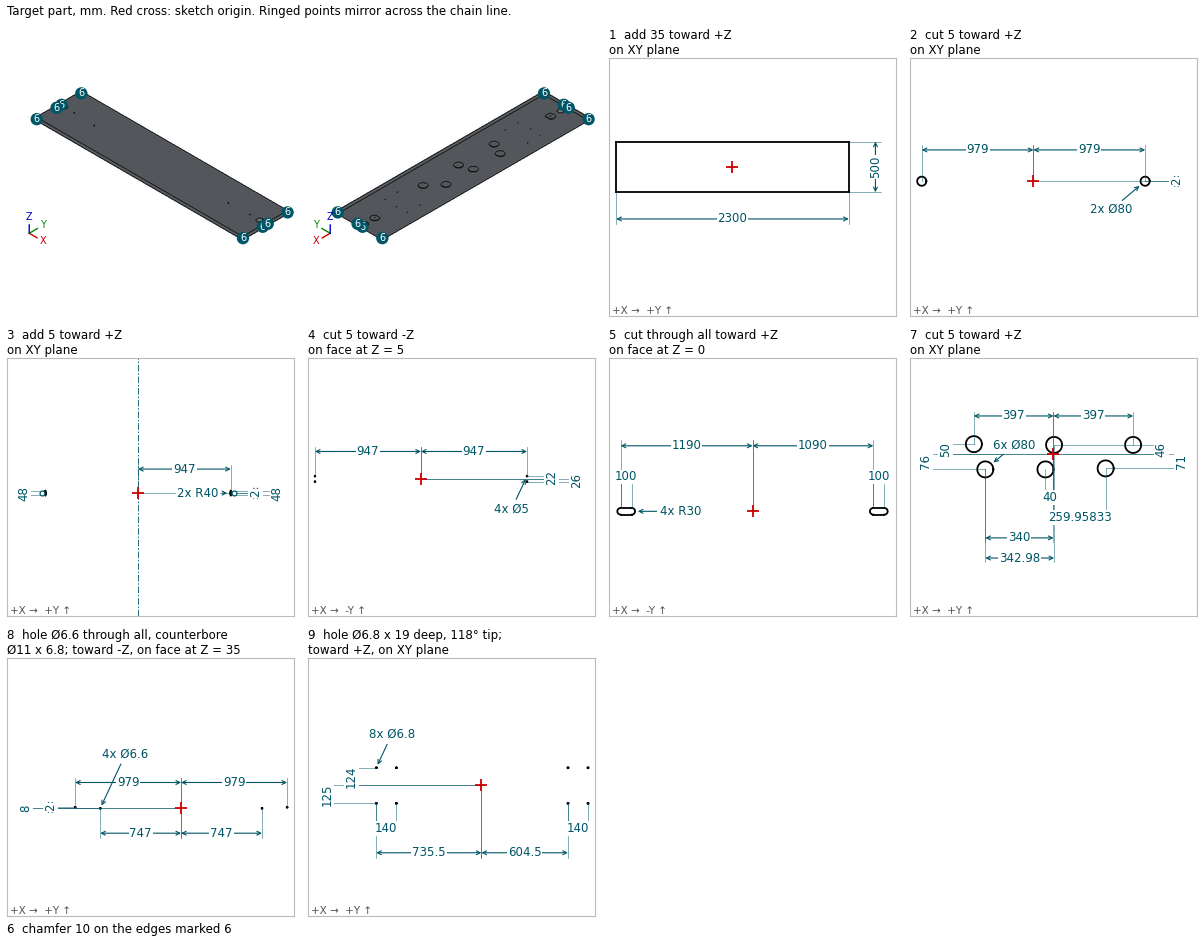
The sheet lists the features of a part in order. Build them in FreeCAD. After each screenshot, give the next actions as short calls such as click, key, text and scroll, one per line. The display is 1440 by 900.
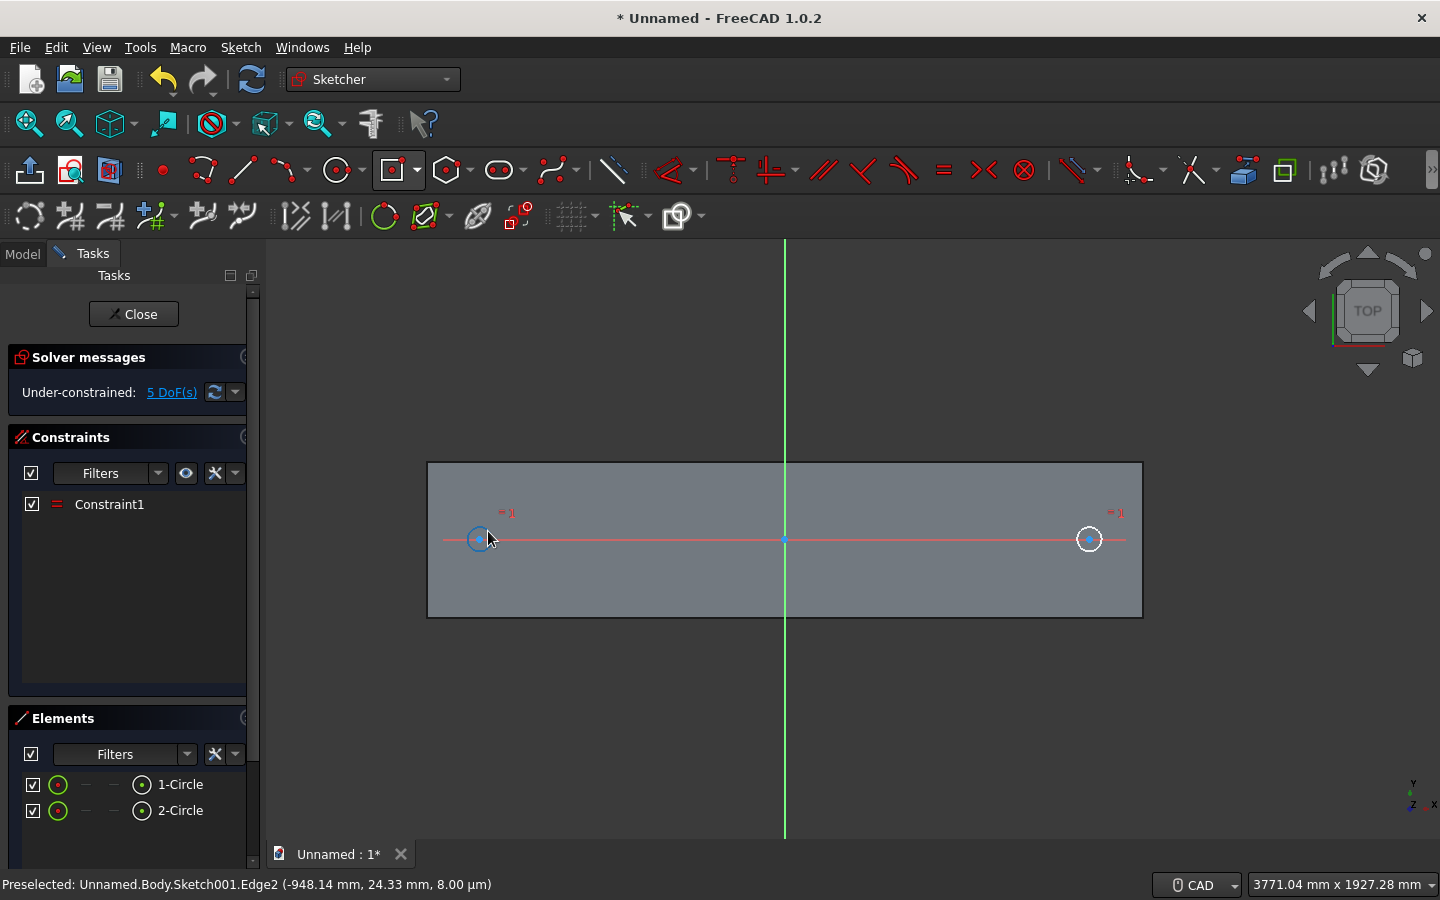
click(1089, 539)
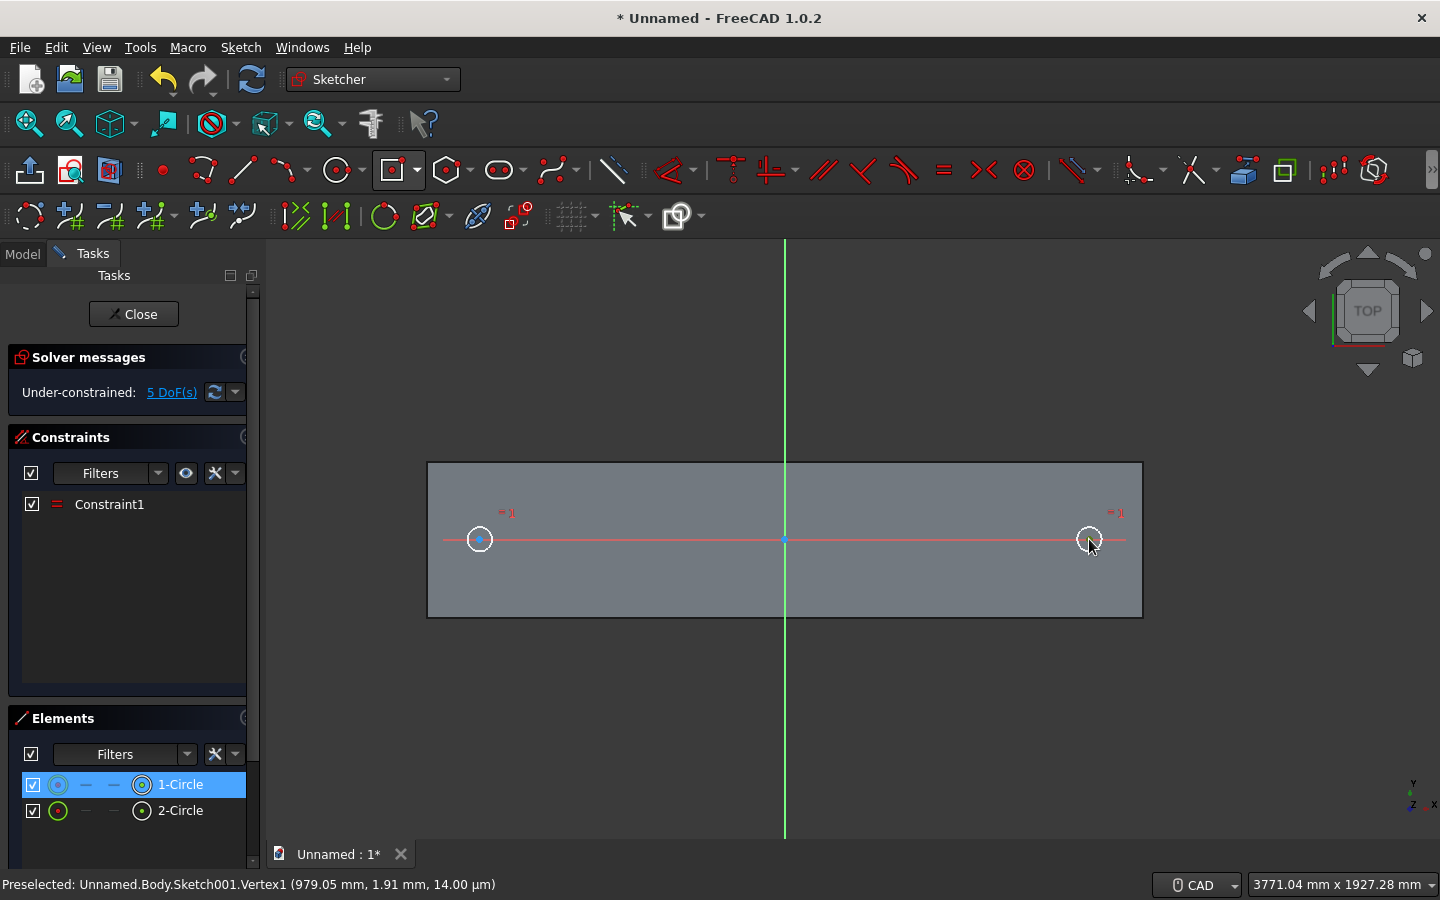
click(480, 539)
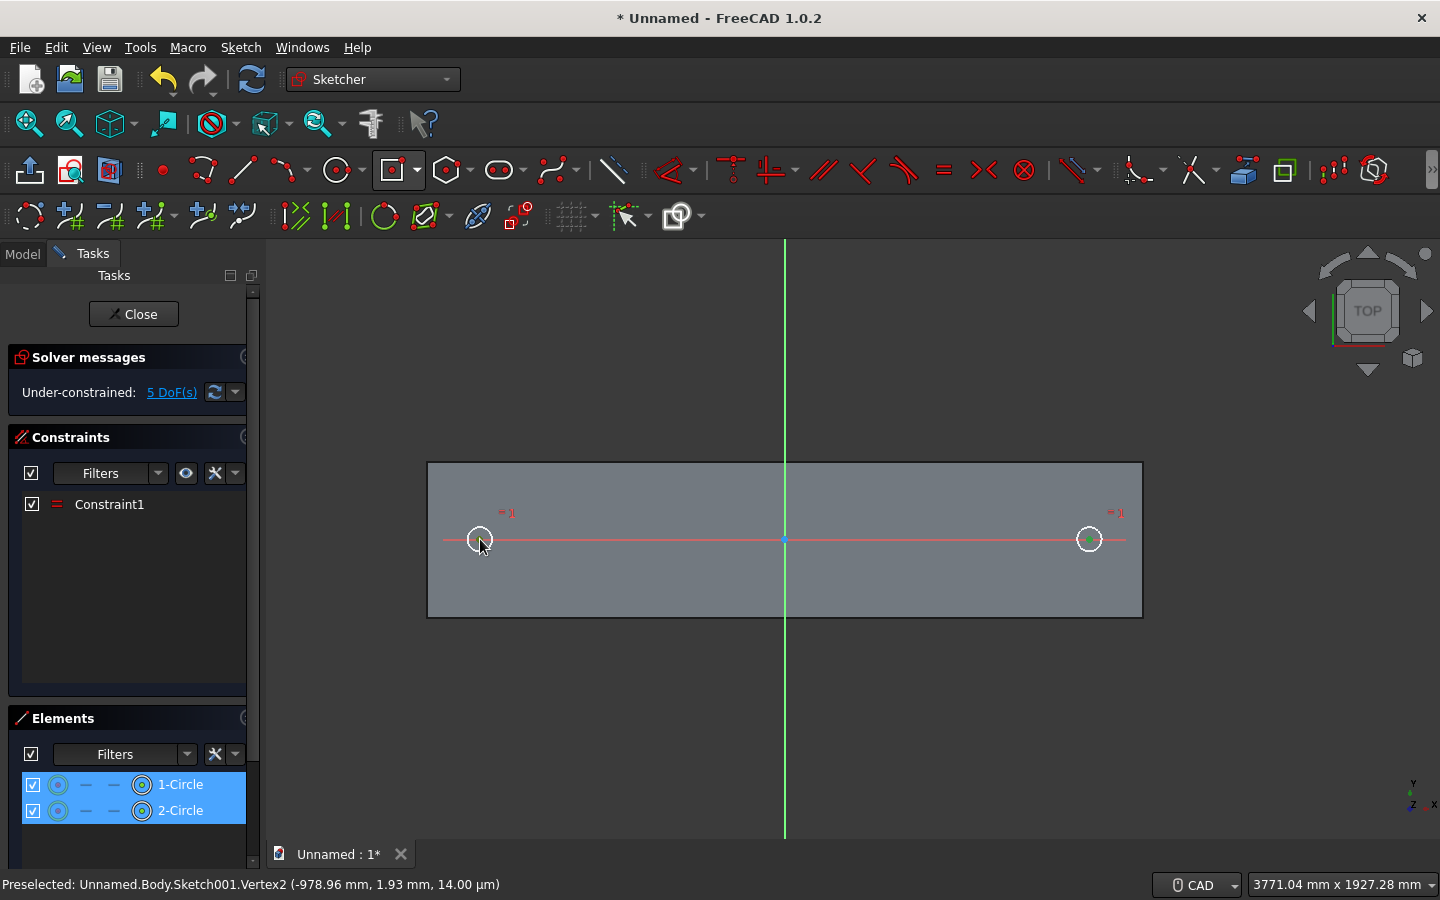
key(h)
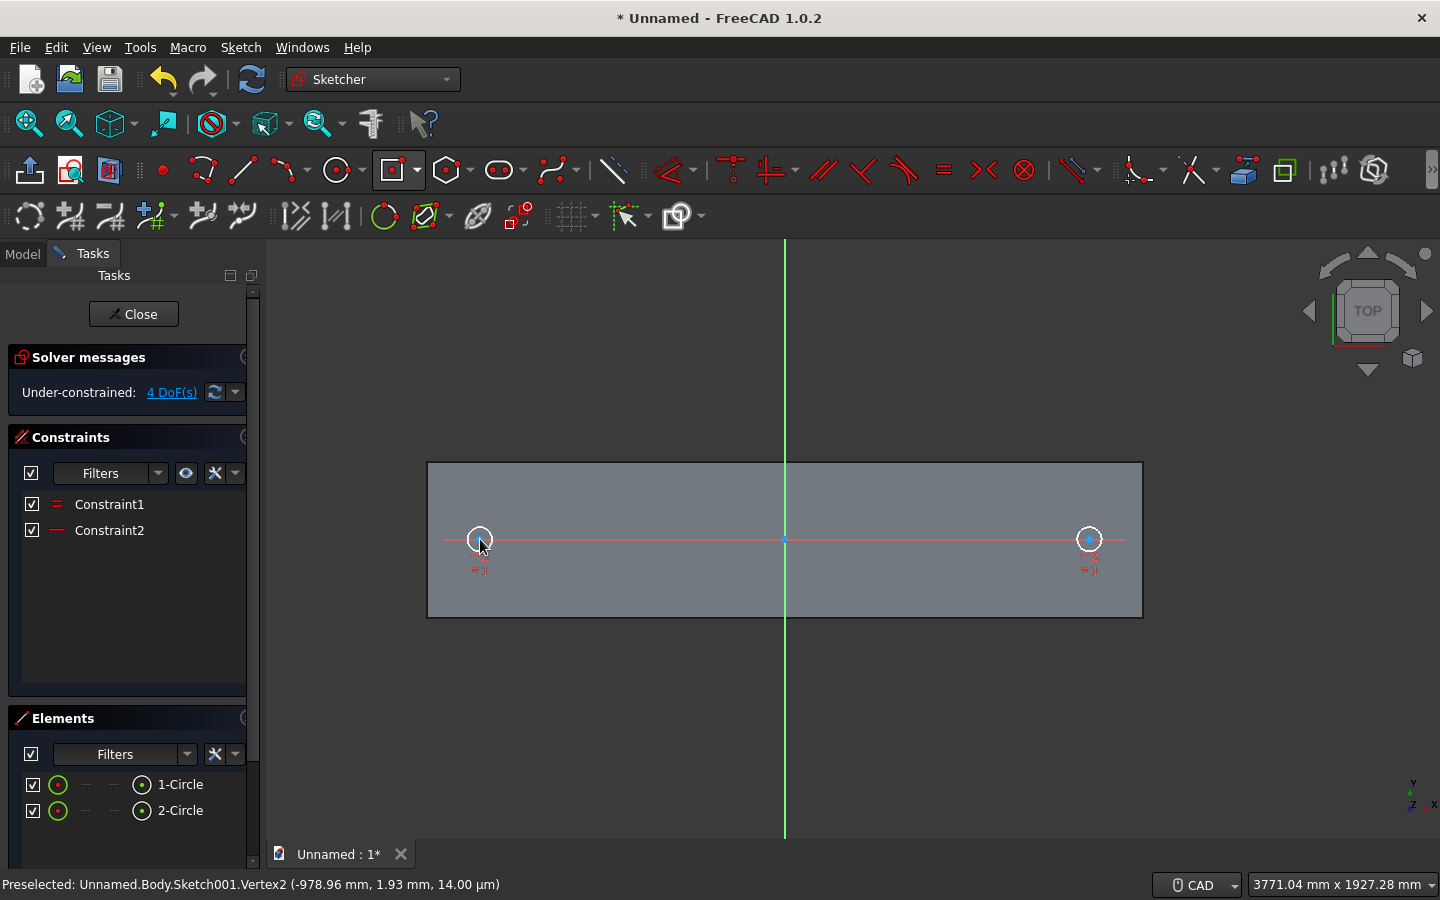
click(668, 170)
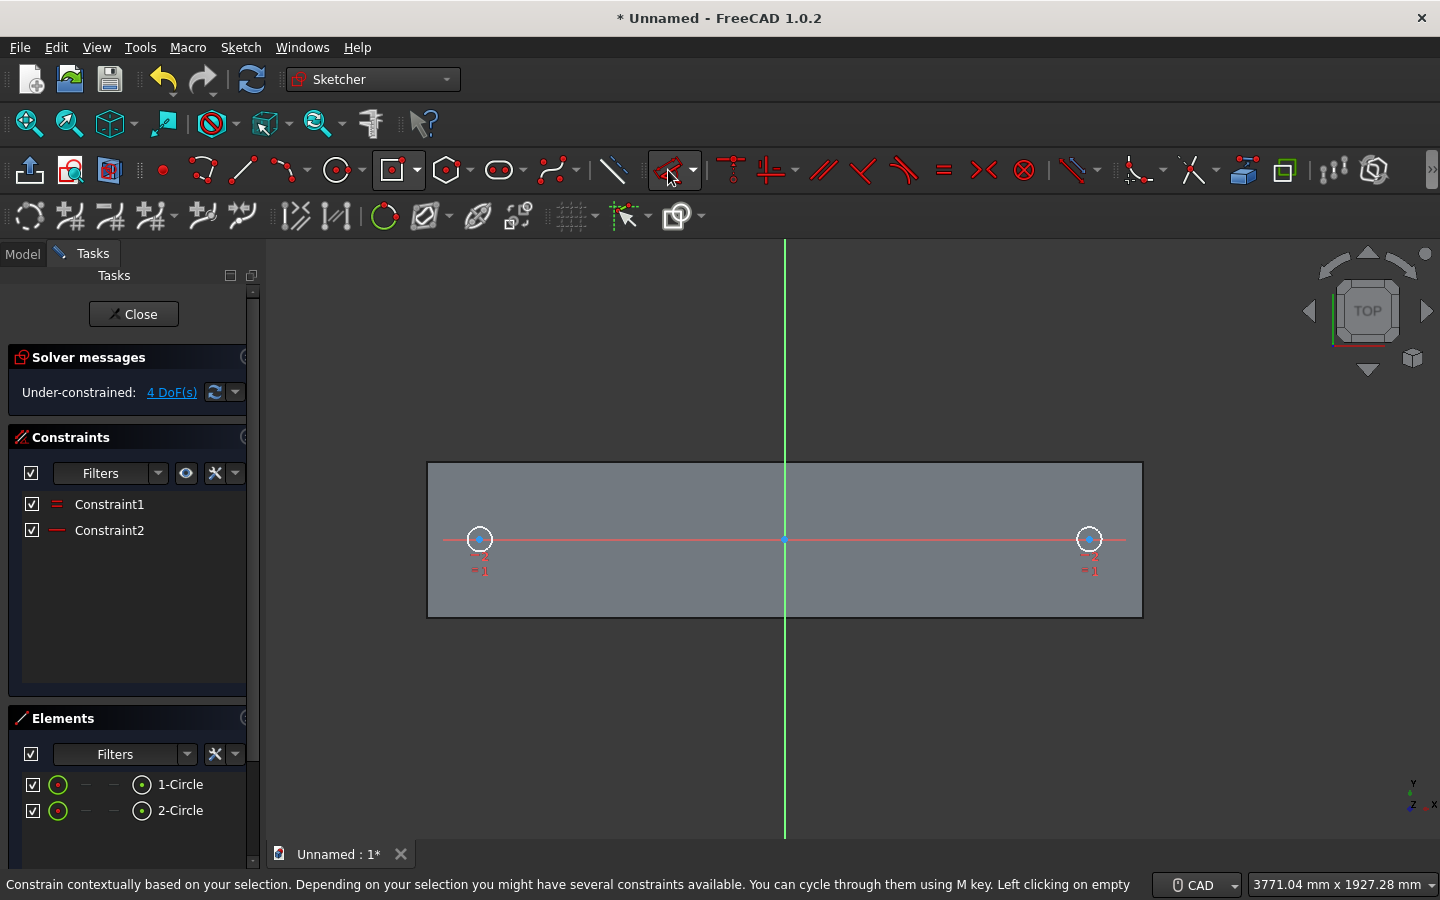
scroll(1098, 531, up, 3)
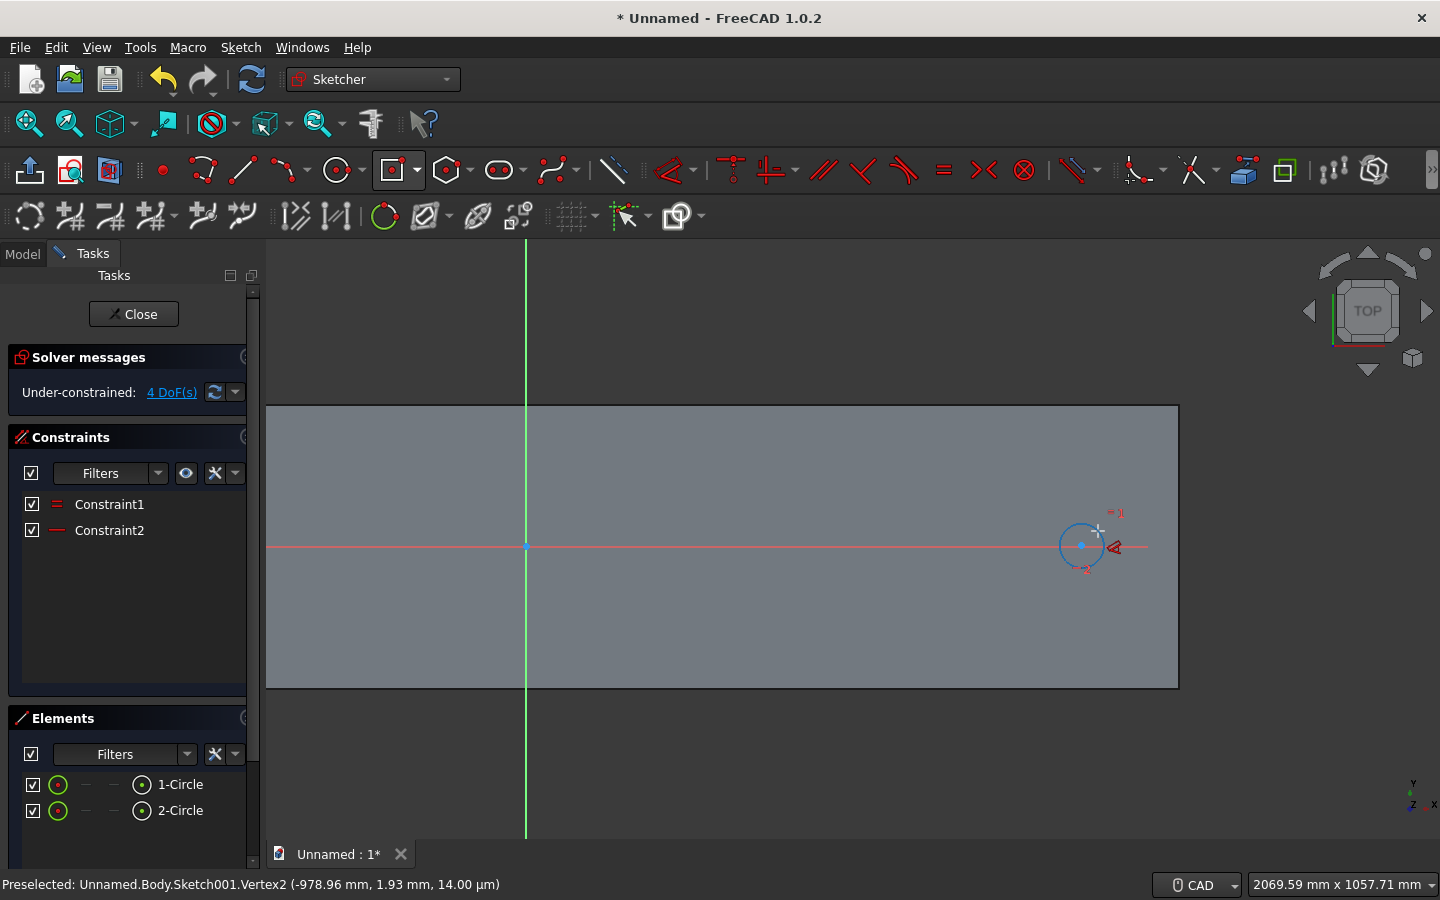
click(1097, 530)
click(1119, 507)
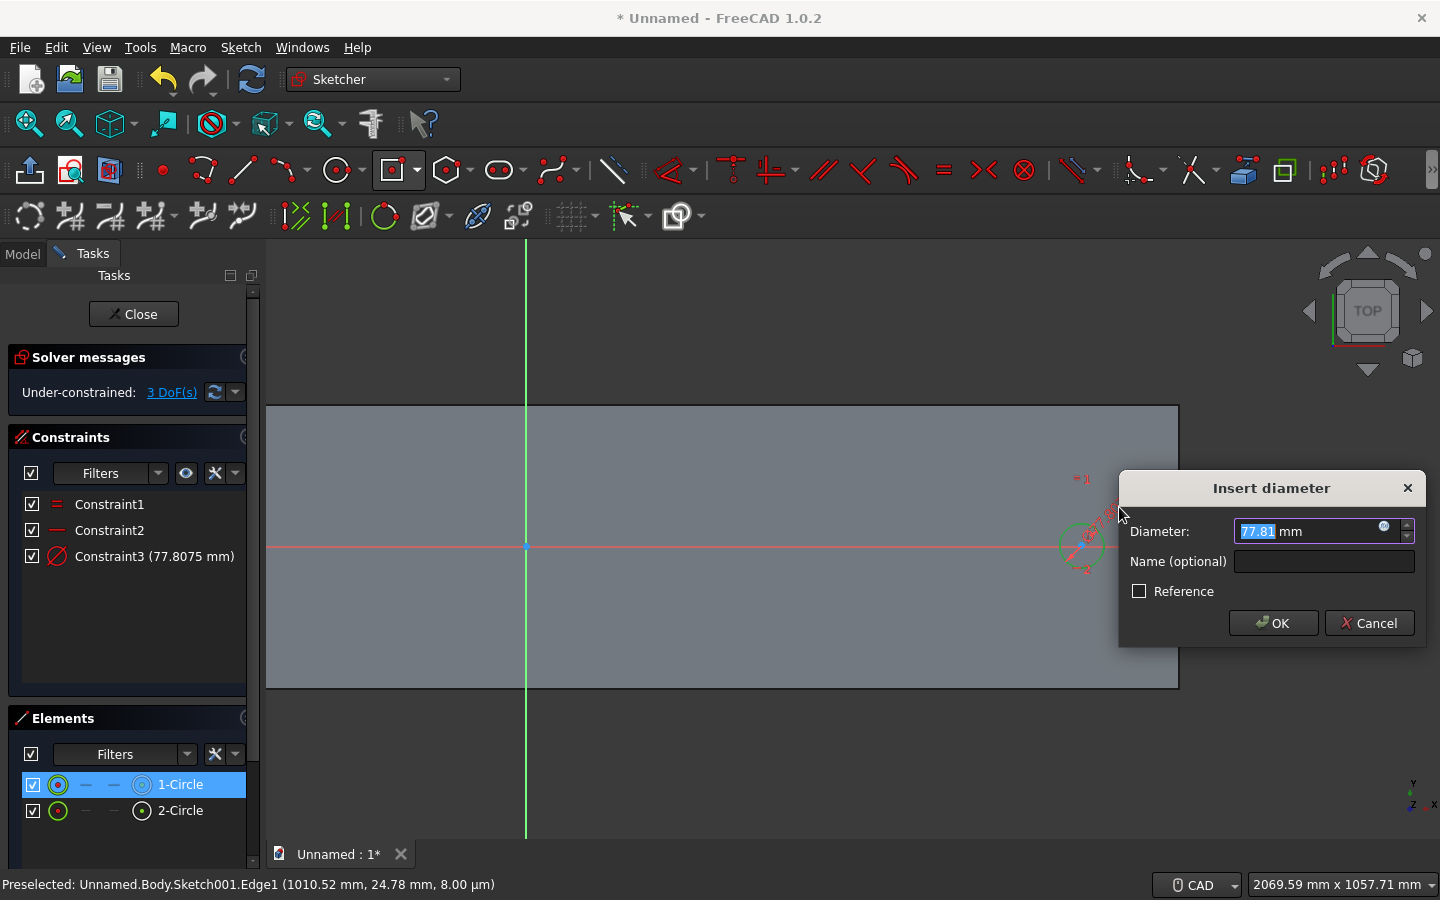
text(80)
key(Return)